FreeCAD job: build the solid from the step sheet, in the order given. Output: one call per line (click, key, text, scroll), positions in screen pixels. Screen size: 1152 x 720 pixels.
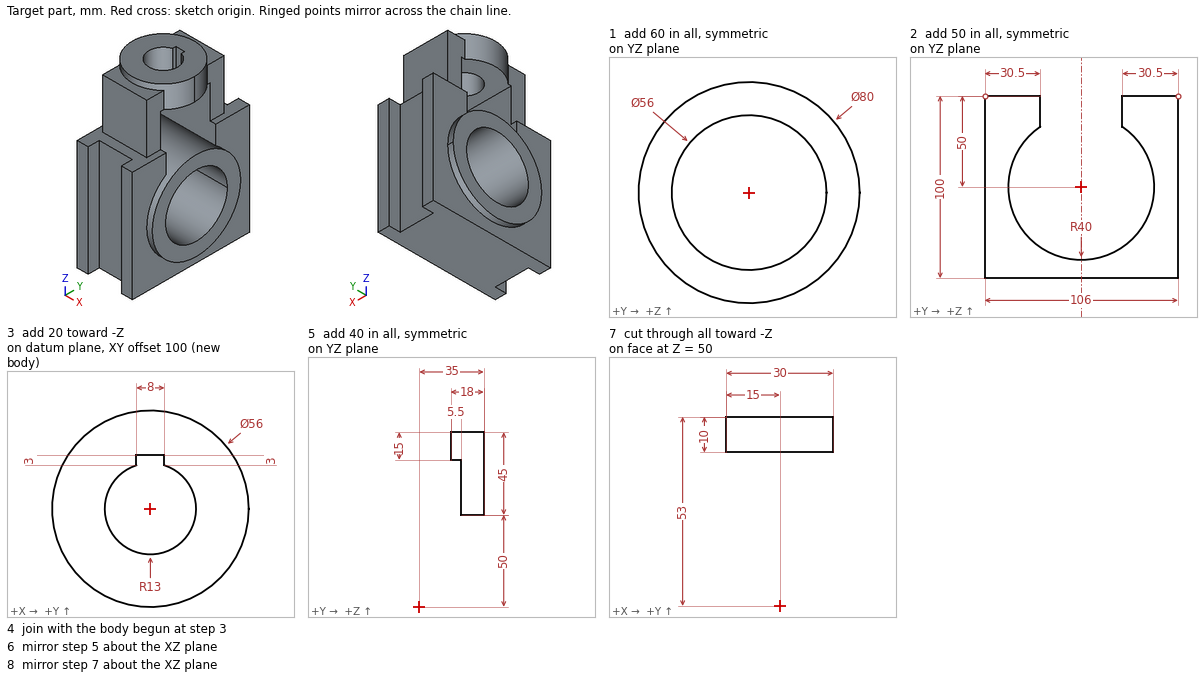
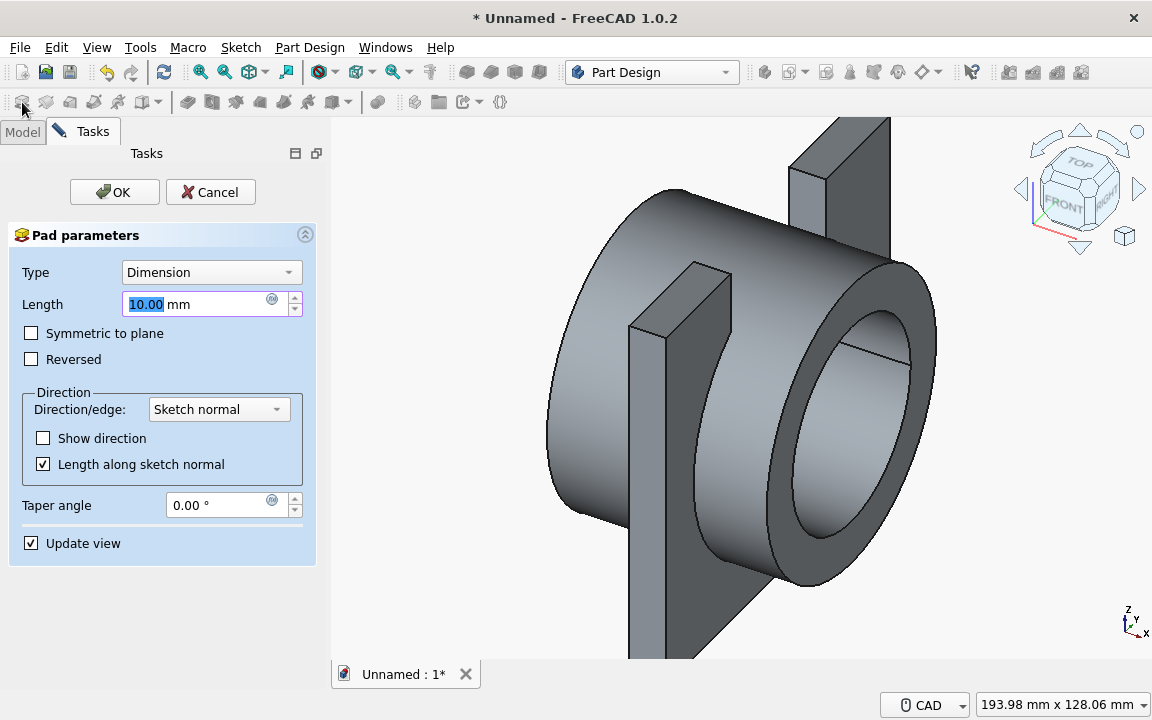
text(50)
key(Tab)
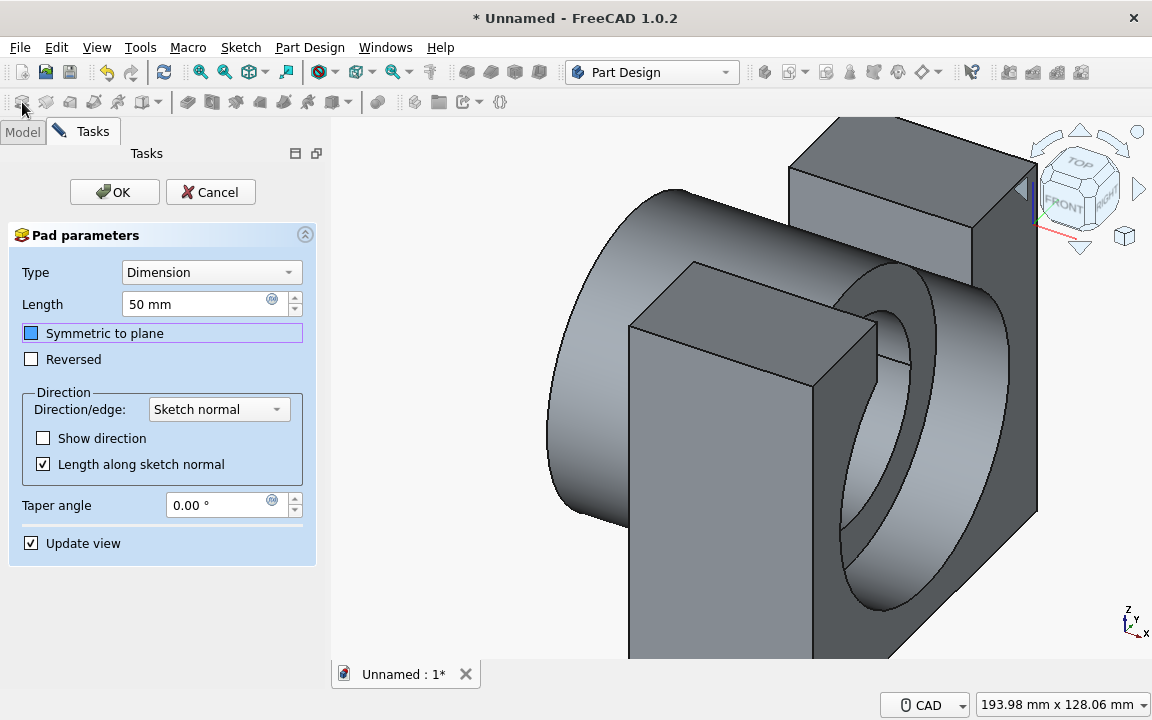
click(30, 333)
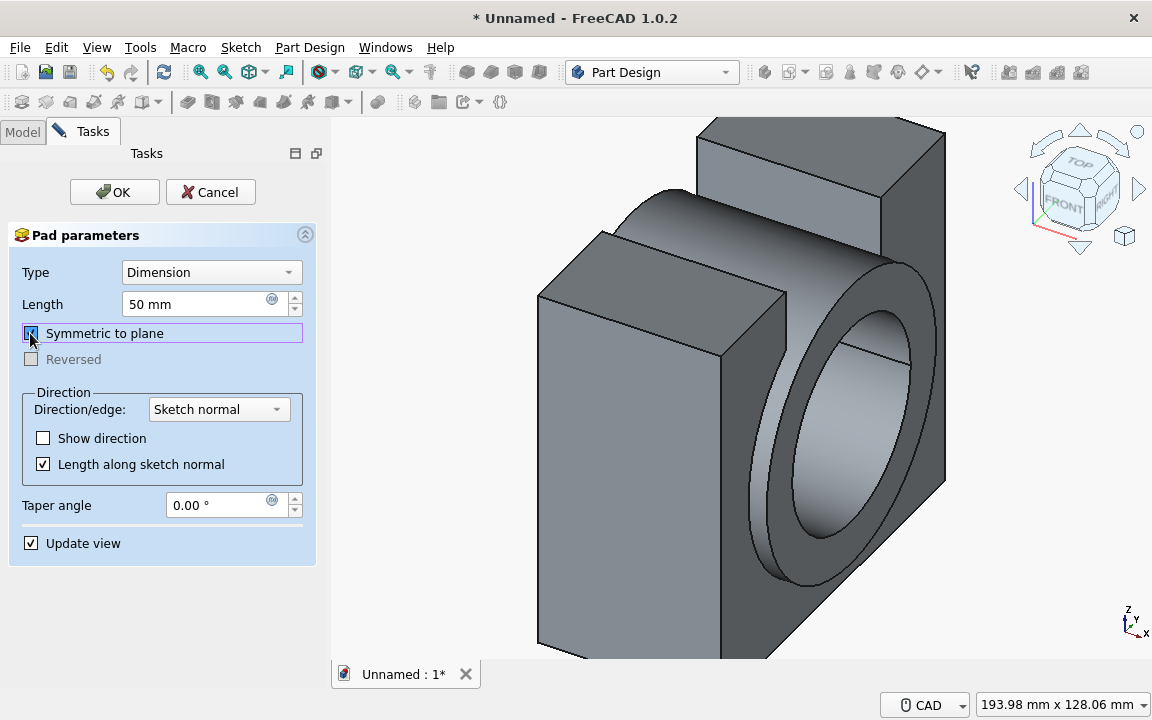
click(115, 192)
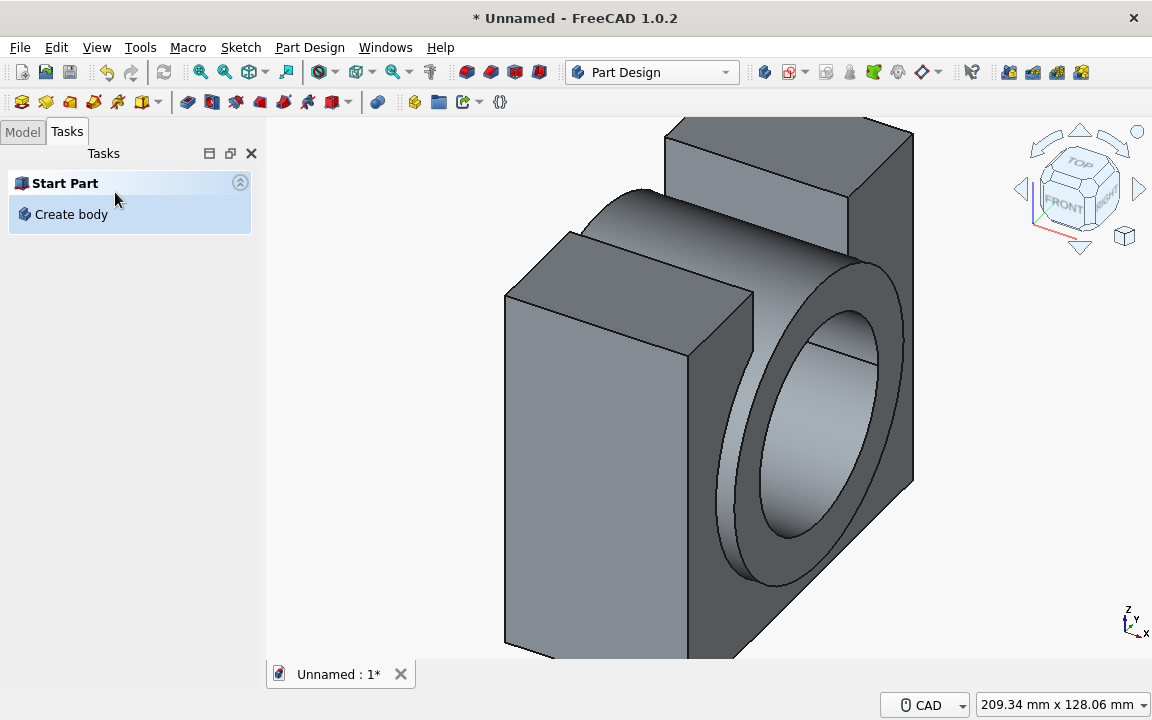
click(202, 72)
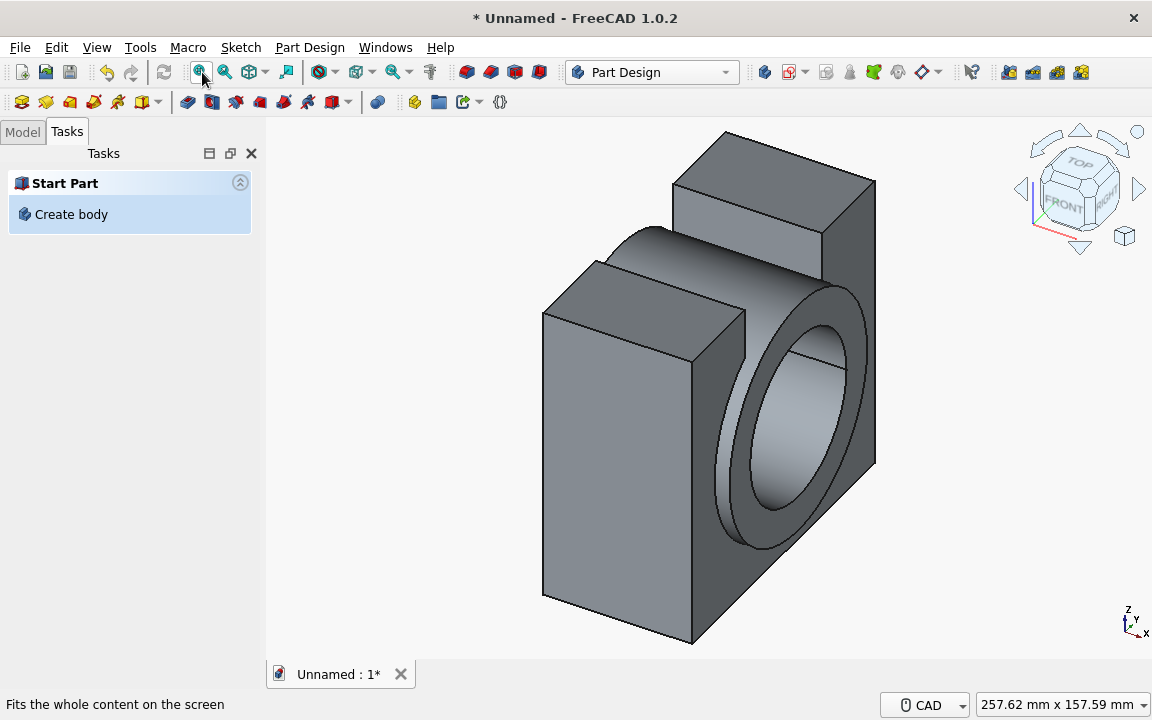
click(766, 72)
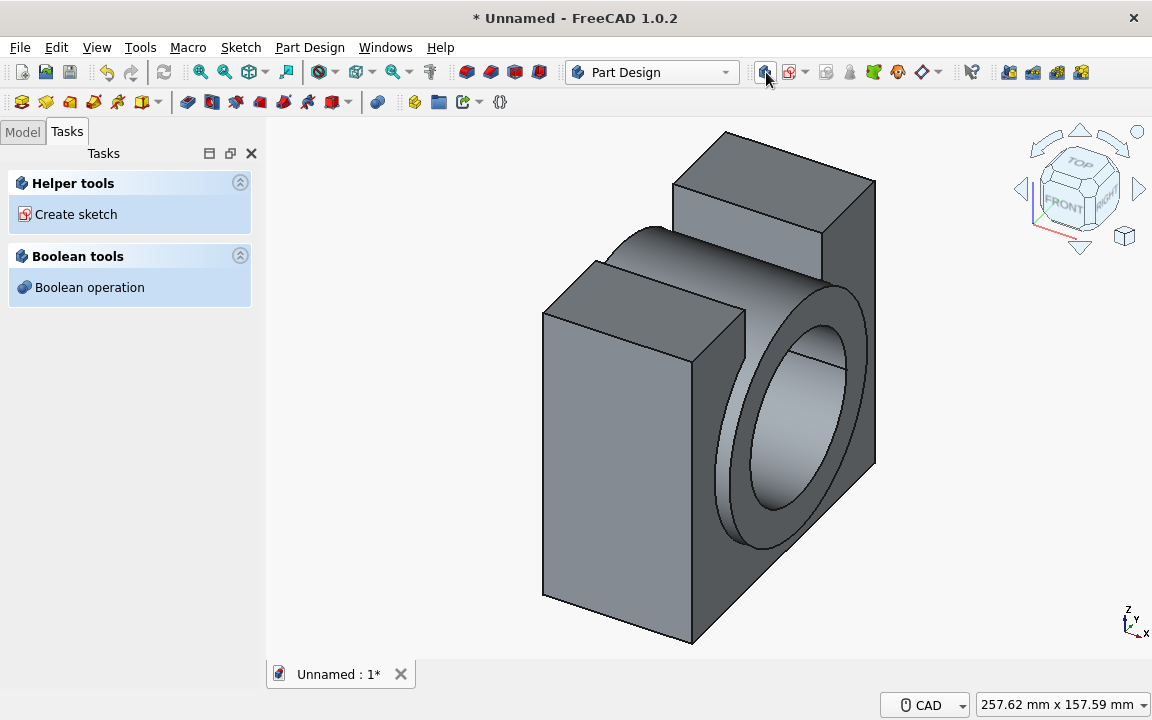
click(23, 131)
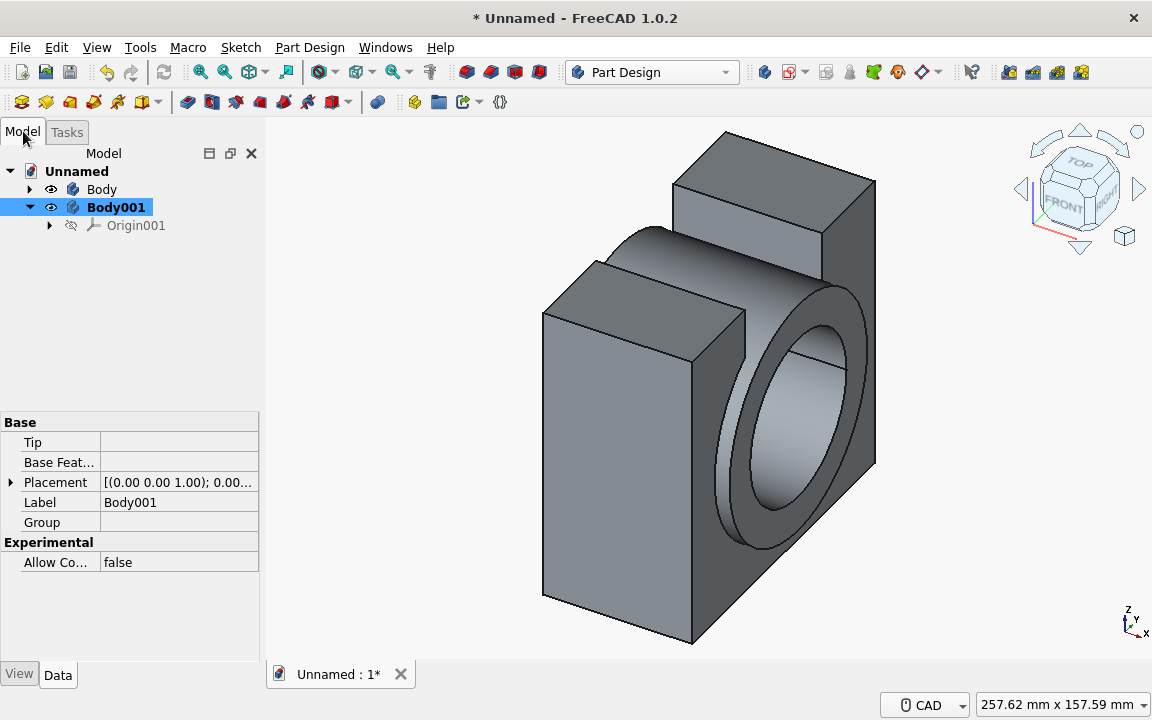
click(50, 225)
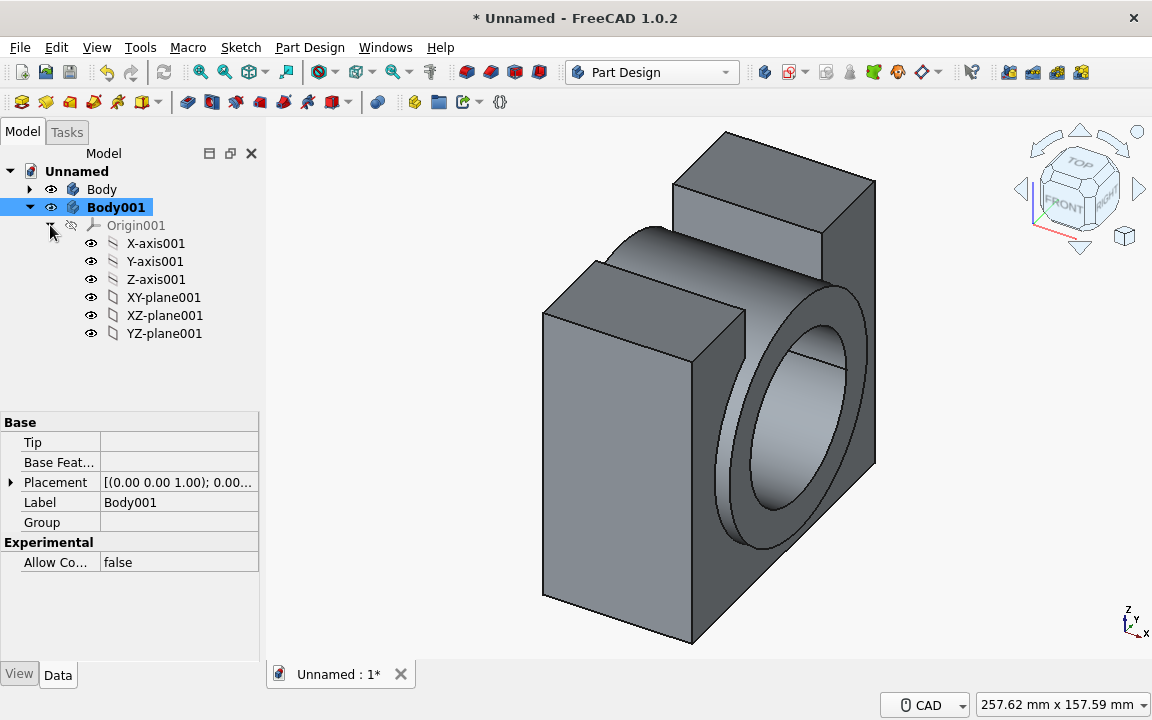
click(136, 297)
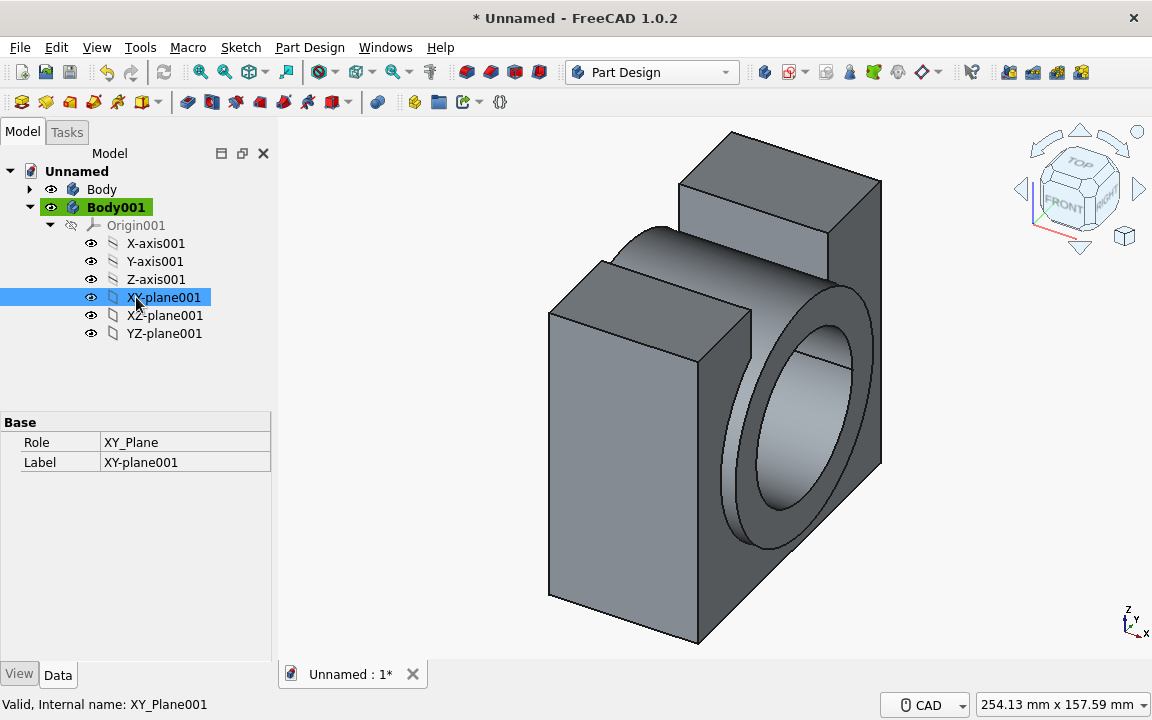
click(922, 72)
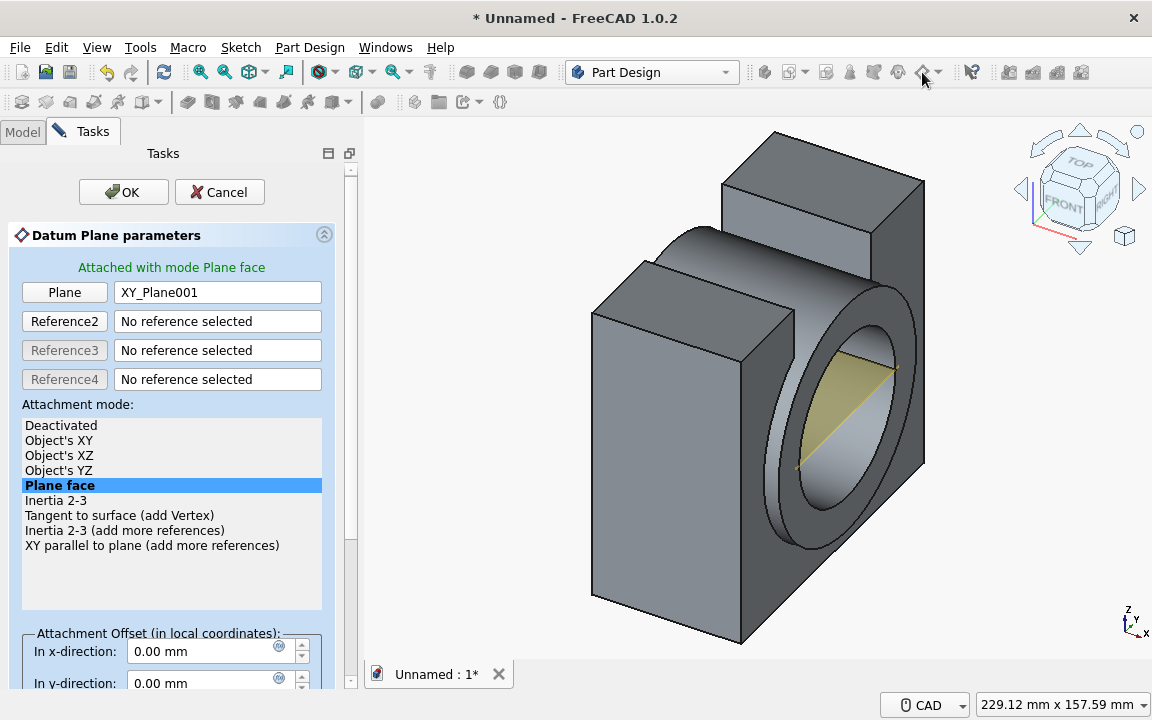
scroll(351, 426, down, 2)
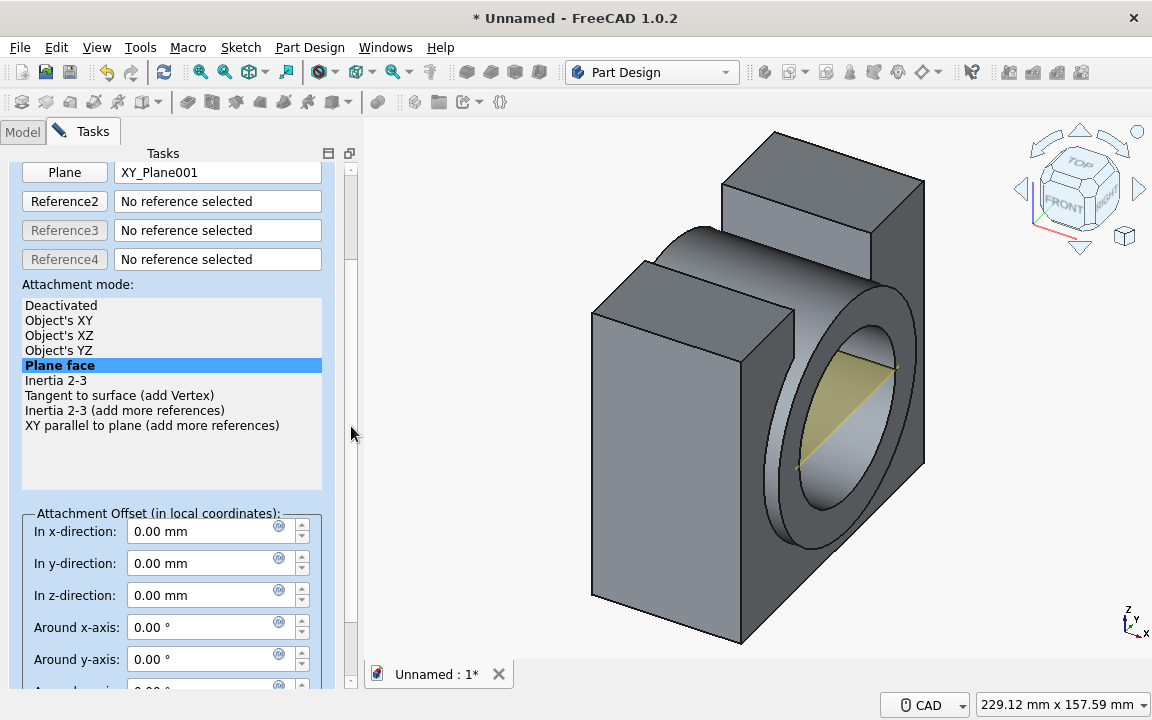
triple_click(210, 595)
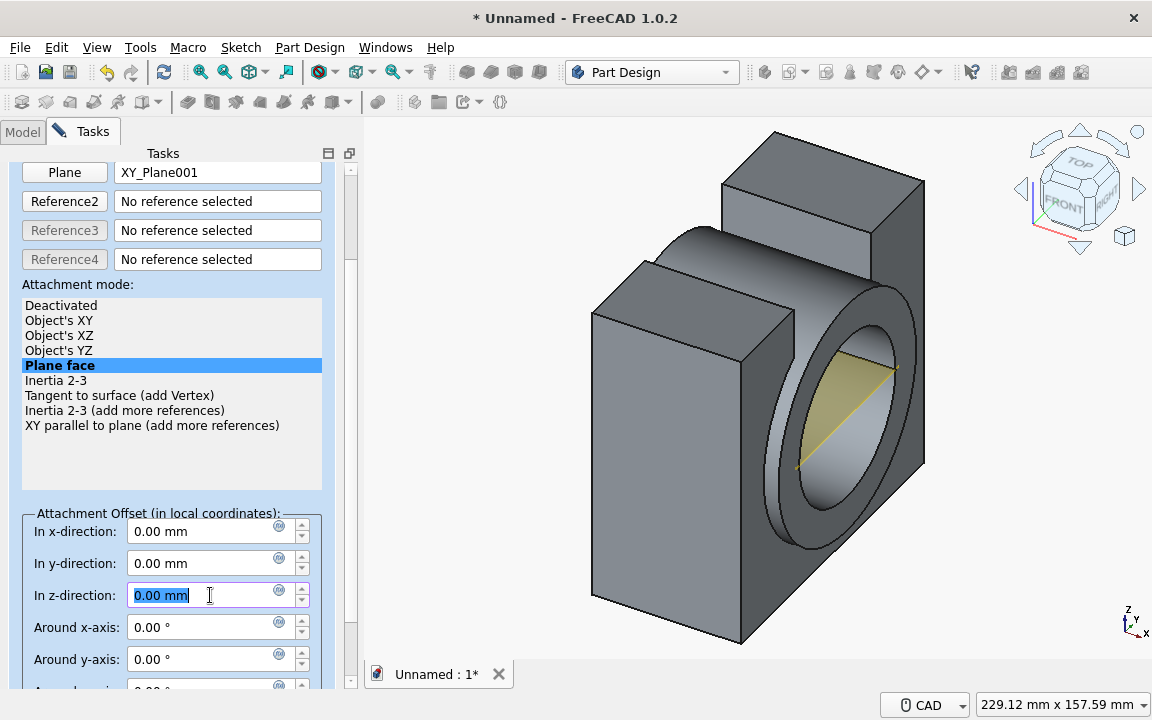
text(100)
key(Tab)